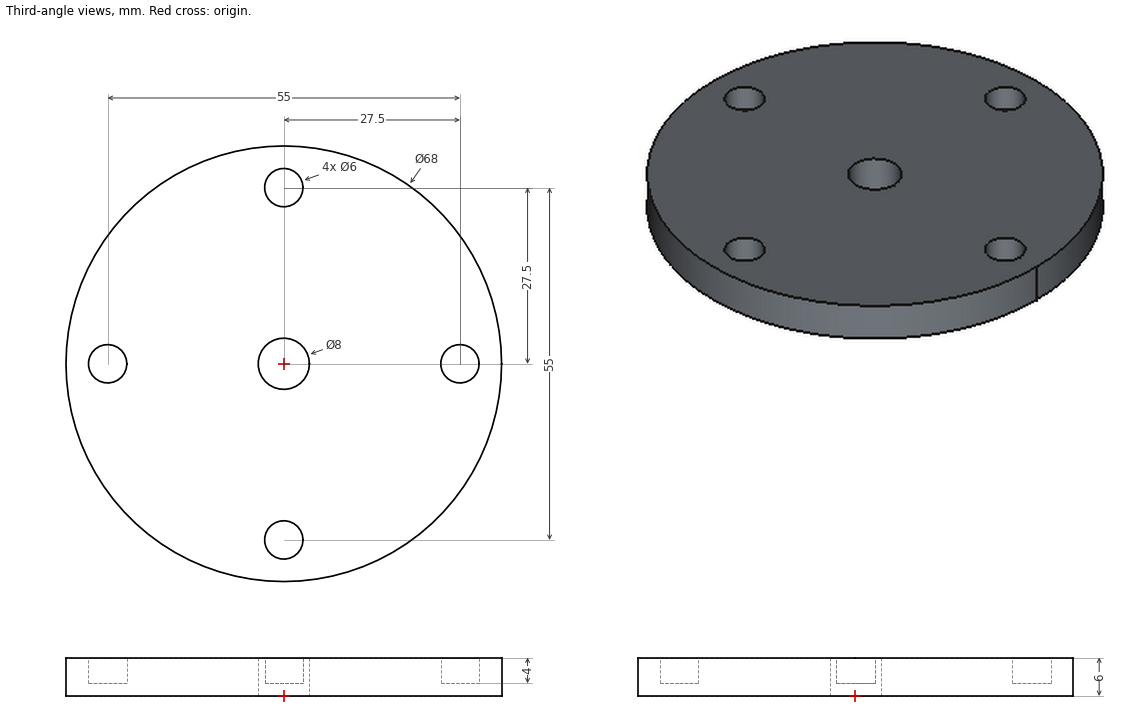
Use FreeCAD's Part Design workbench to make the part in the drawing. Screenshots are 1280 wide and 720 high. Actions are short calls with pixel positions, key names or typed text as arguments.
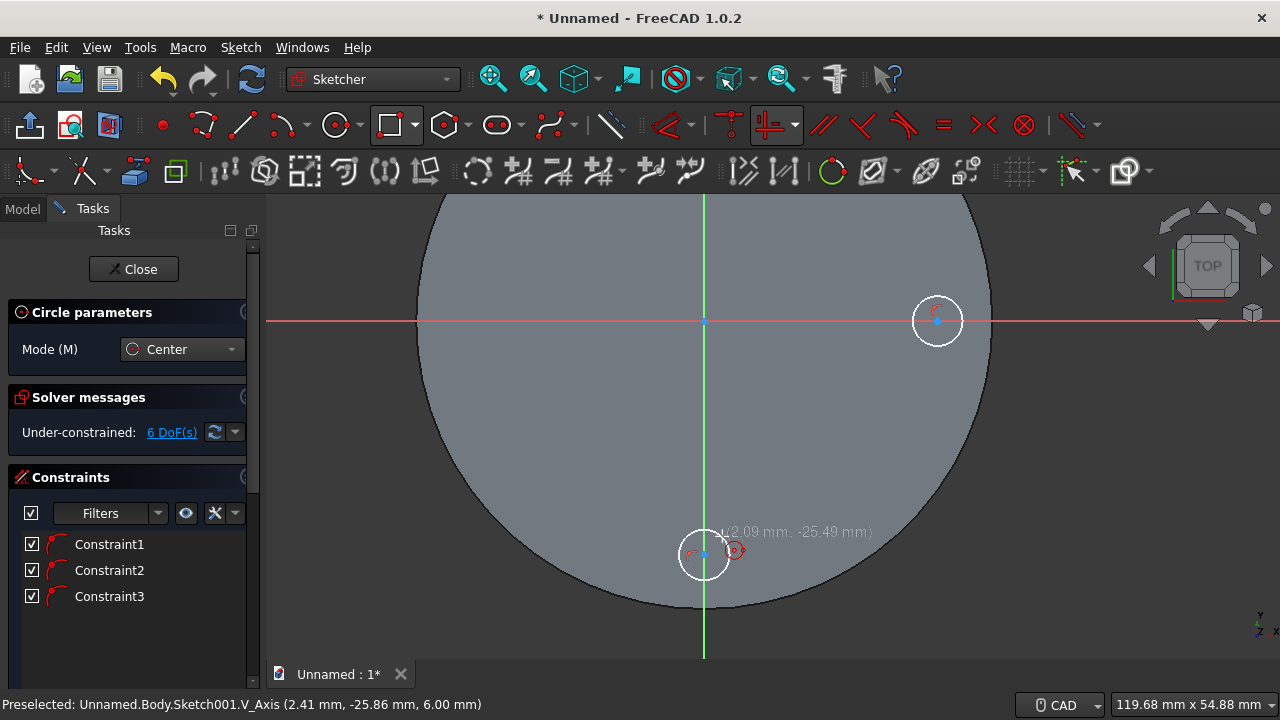
click(471, 321)
click(489, 303)
key(Escape)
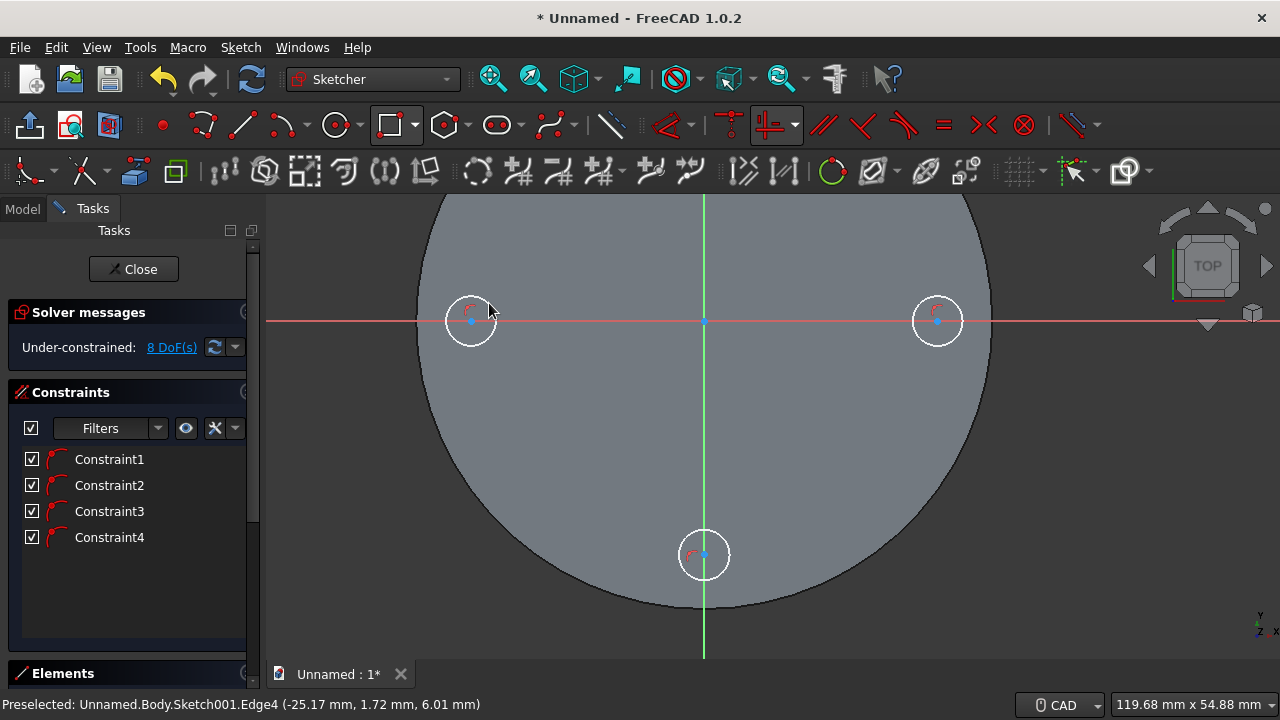
scroll(705, 555, down, 3)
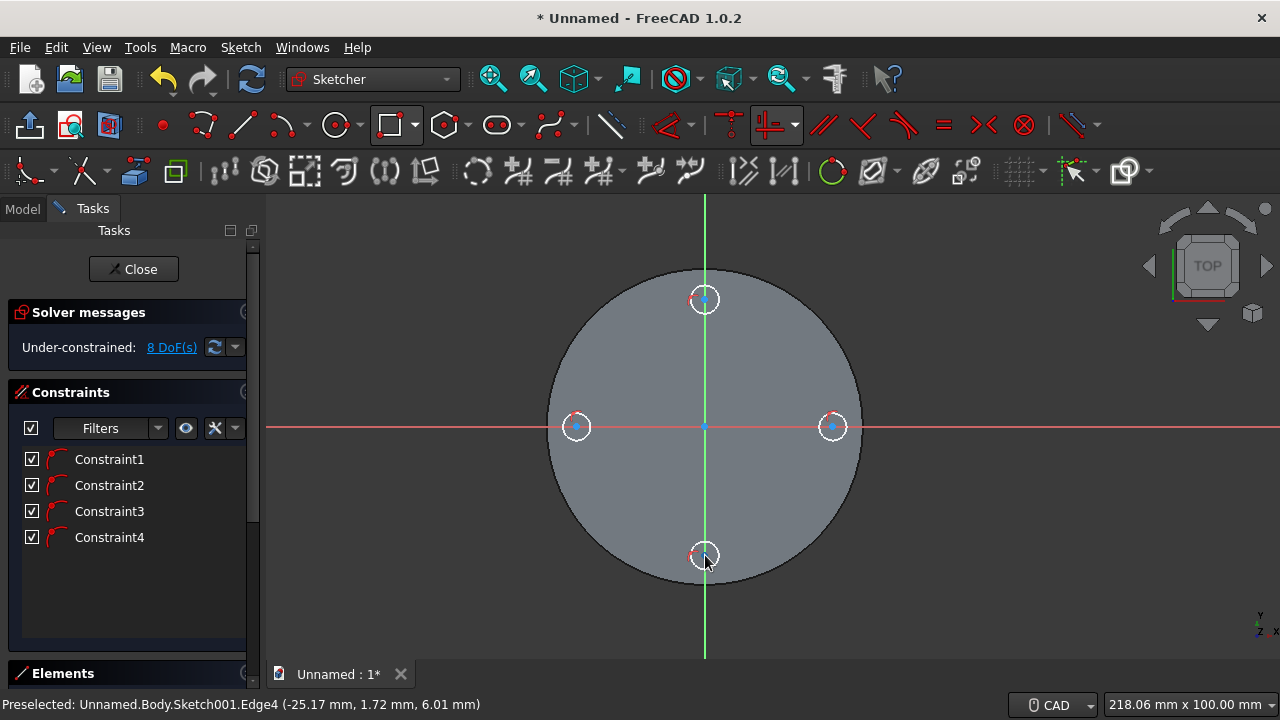
scroll(715, 290, up, 2)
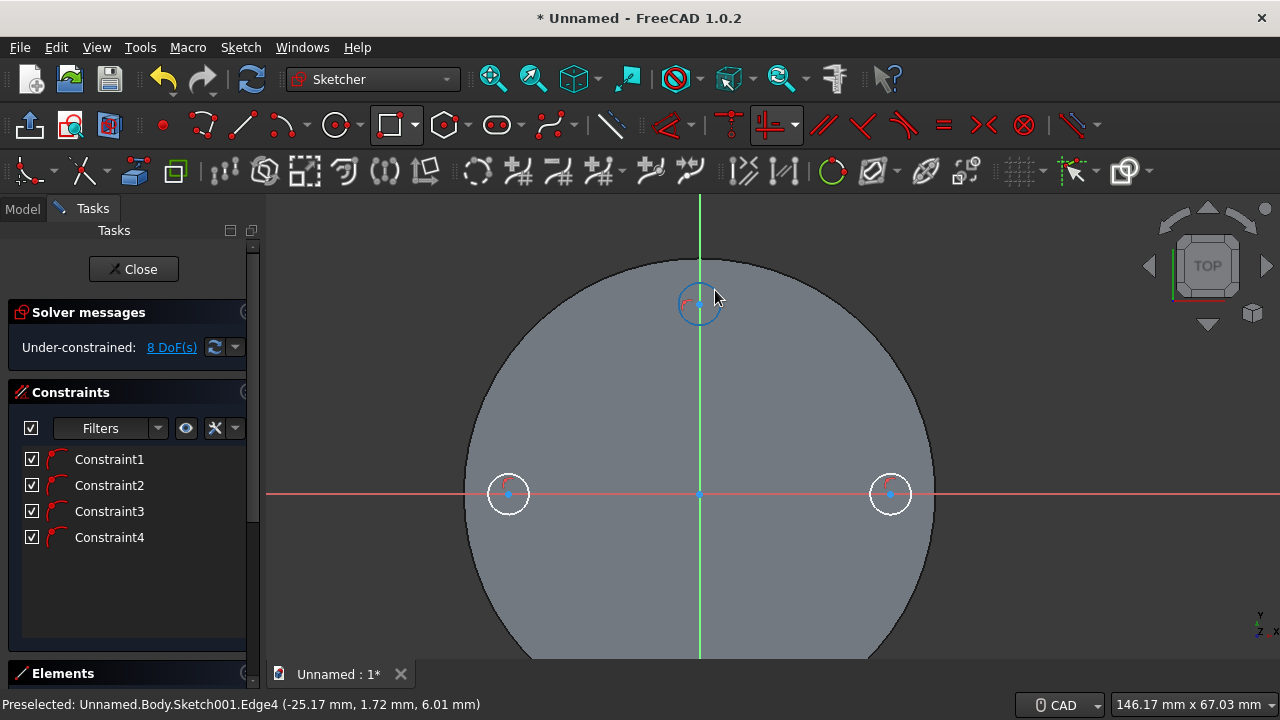
click(714, 289)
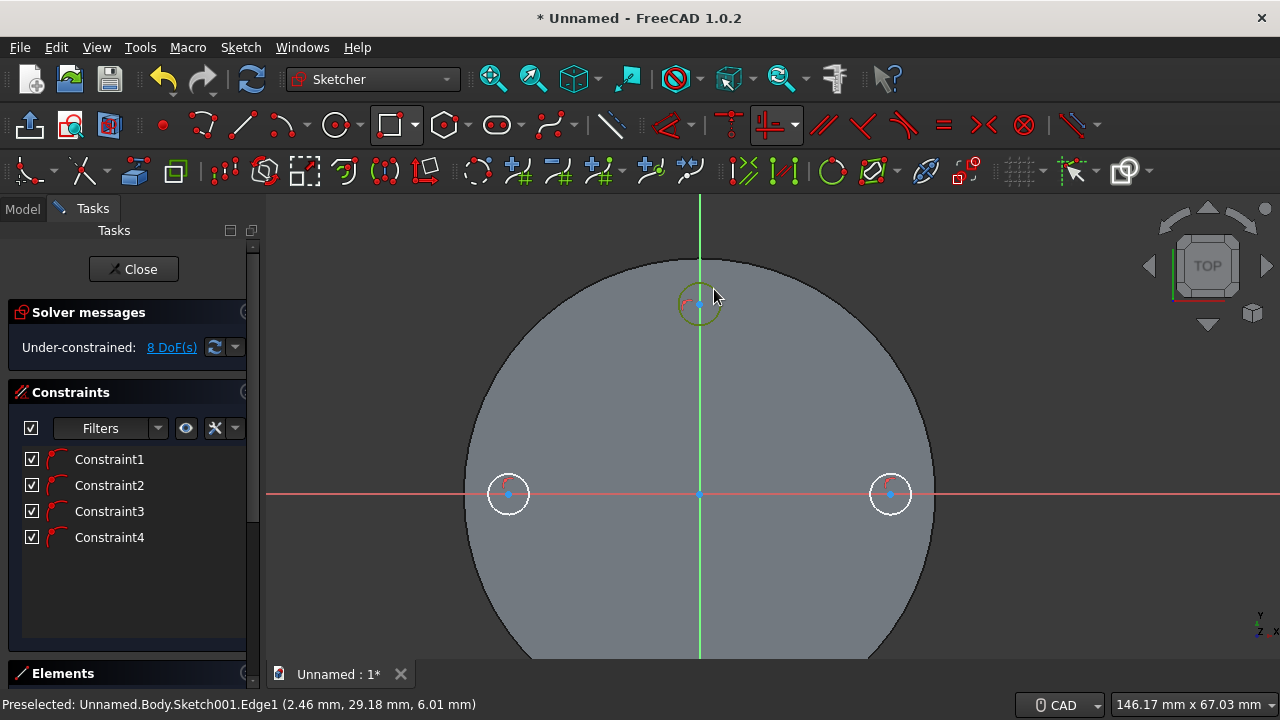
click(905, 480)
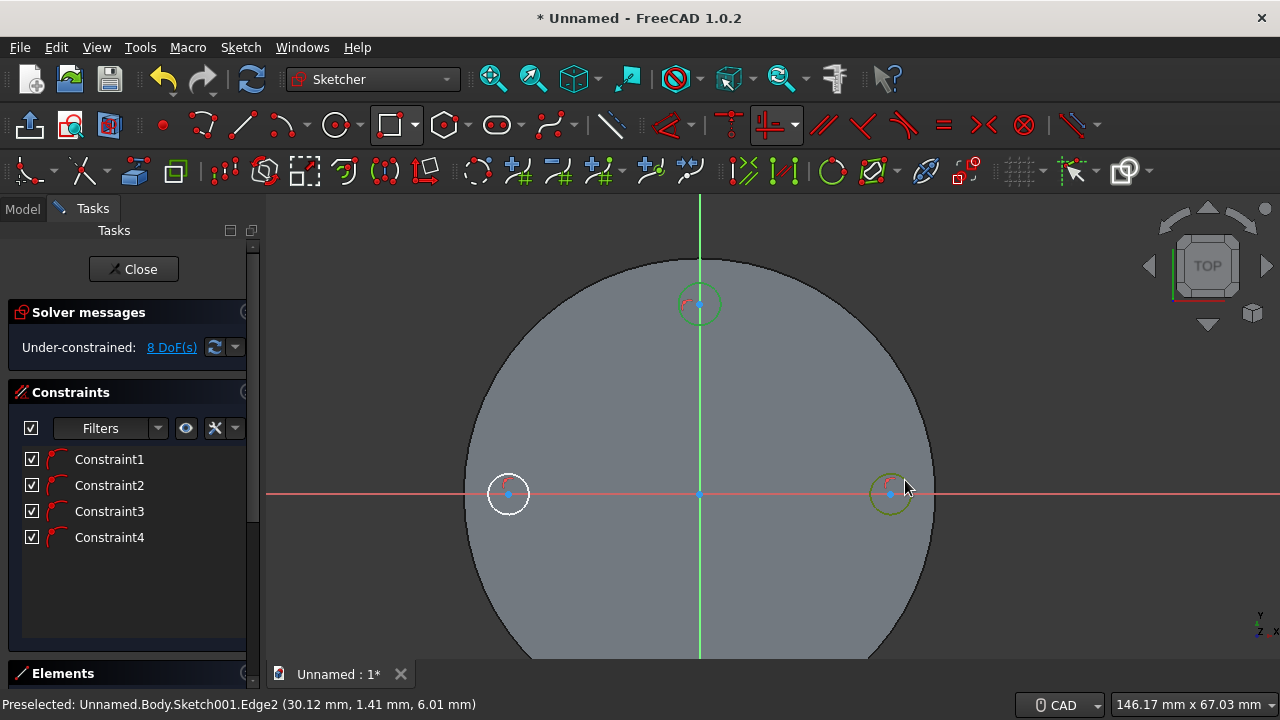
scroll(715, 289, down, 2)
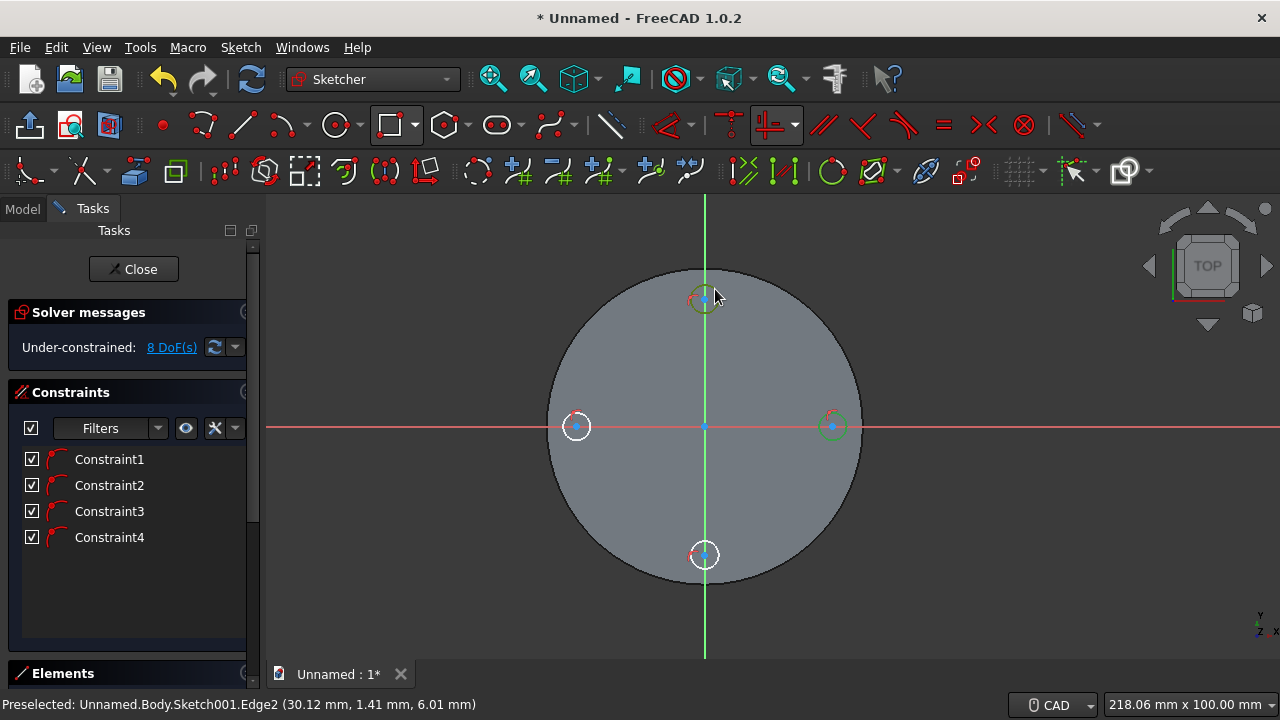
scroll(715, 545, up, 2)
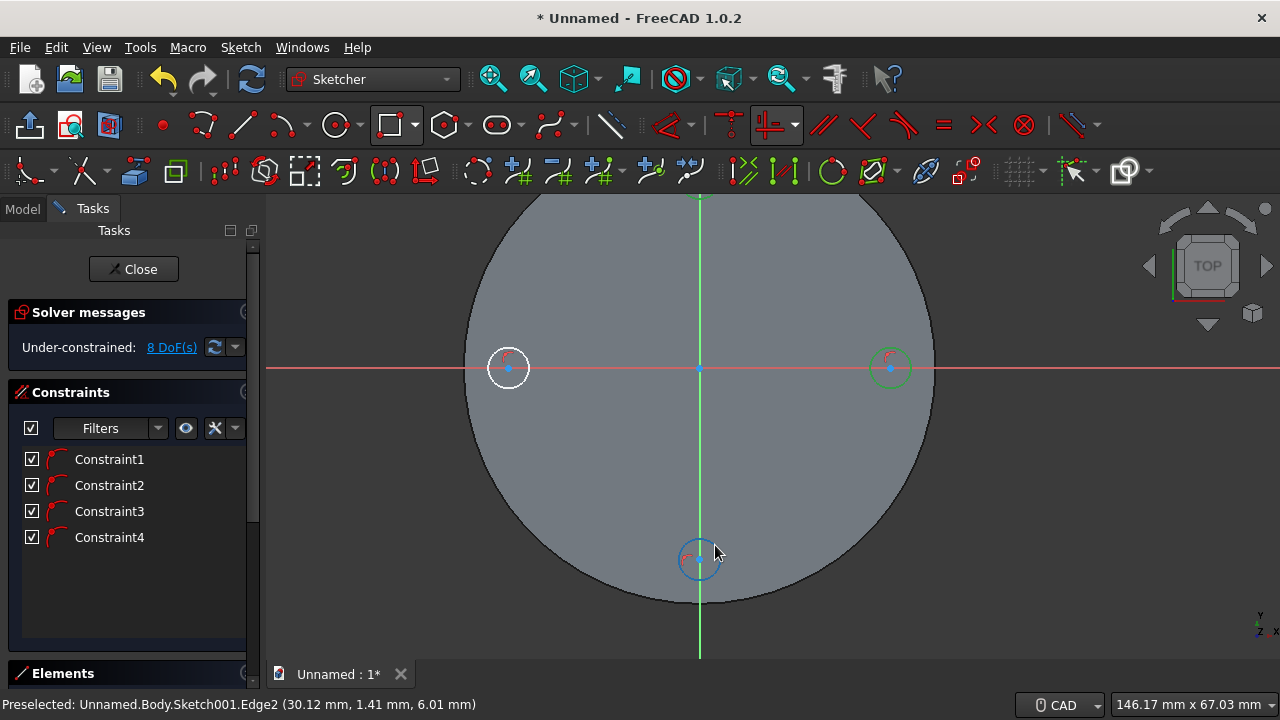
click(714, 545)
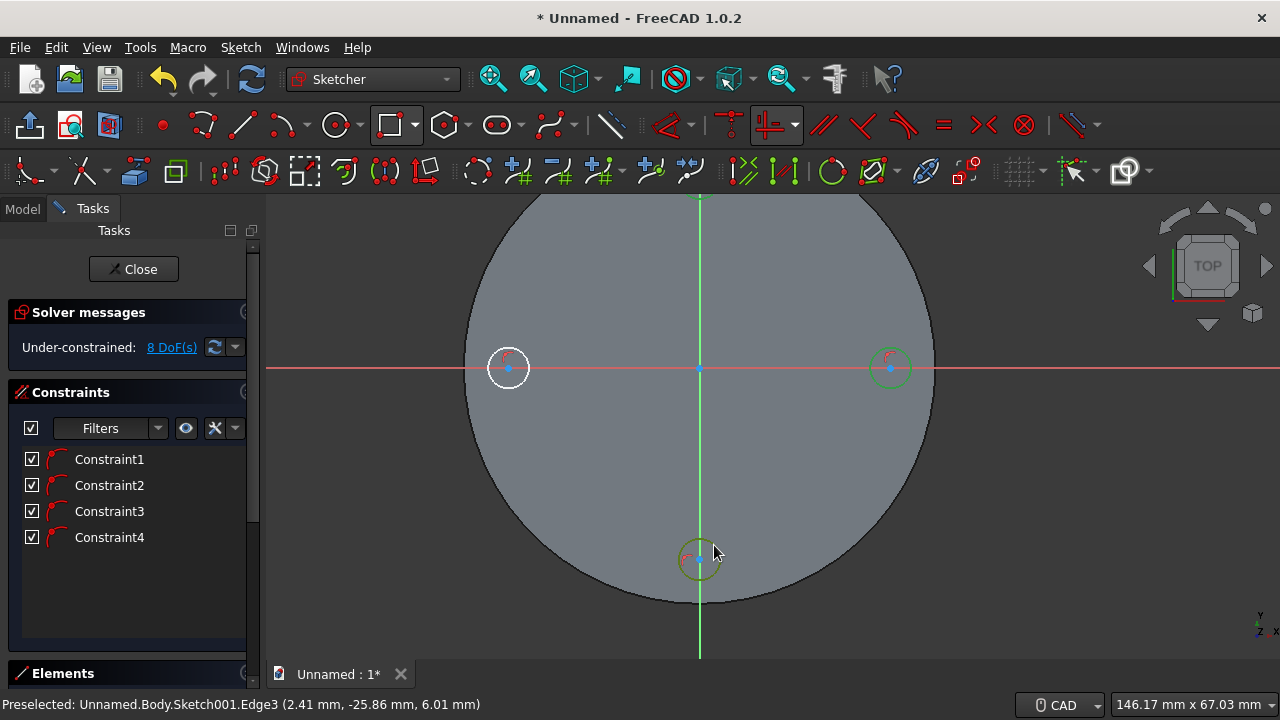
click(523, 354)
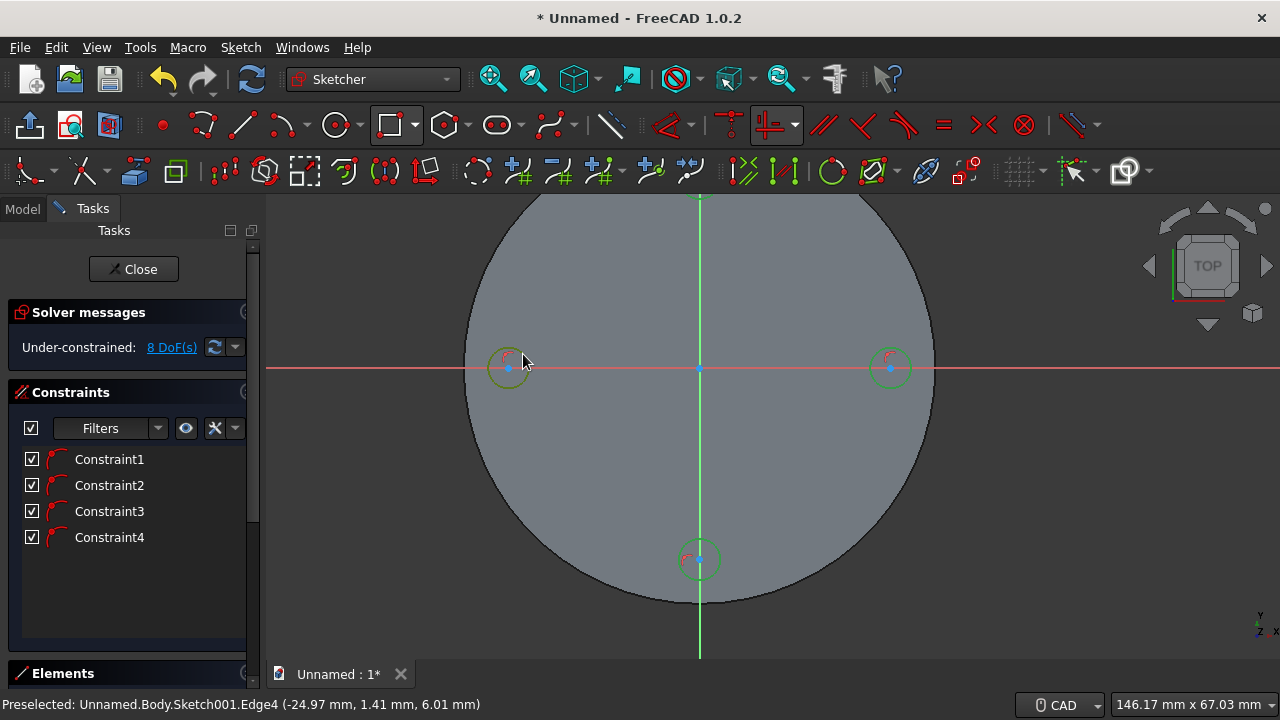
click(944, 126)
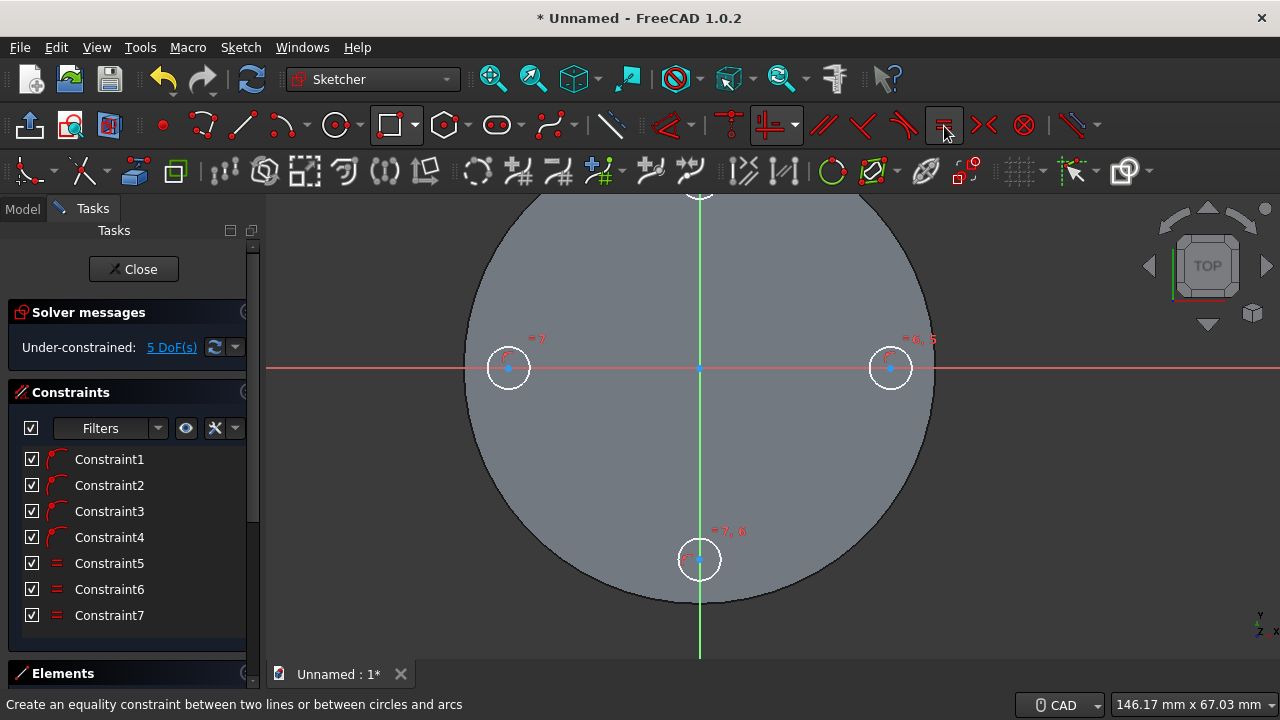
click(666, 126)